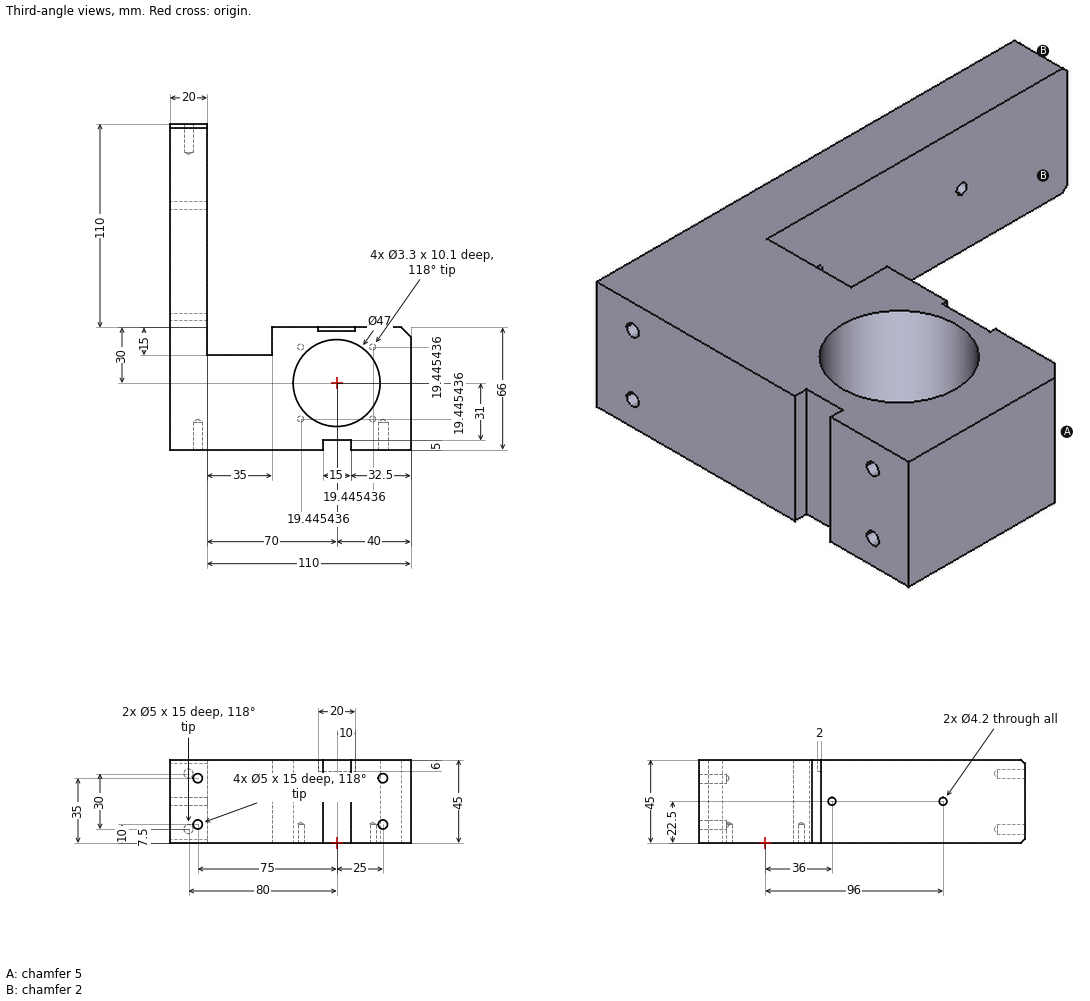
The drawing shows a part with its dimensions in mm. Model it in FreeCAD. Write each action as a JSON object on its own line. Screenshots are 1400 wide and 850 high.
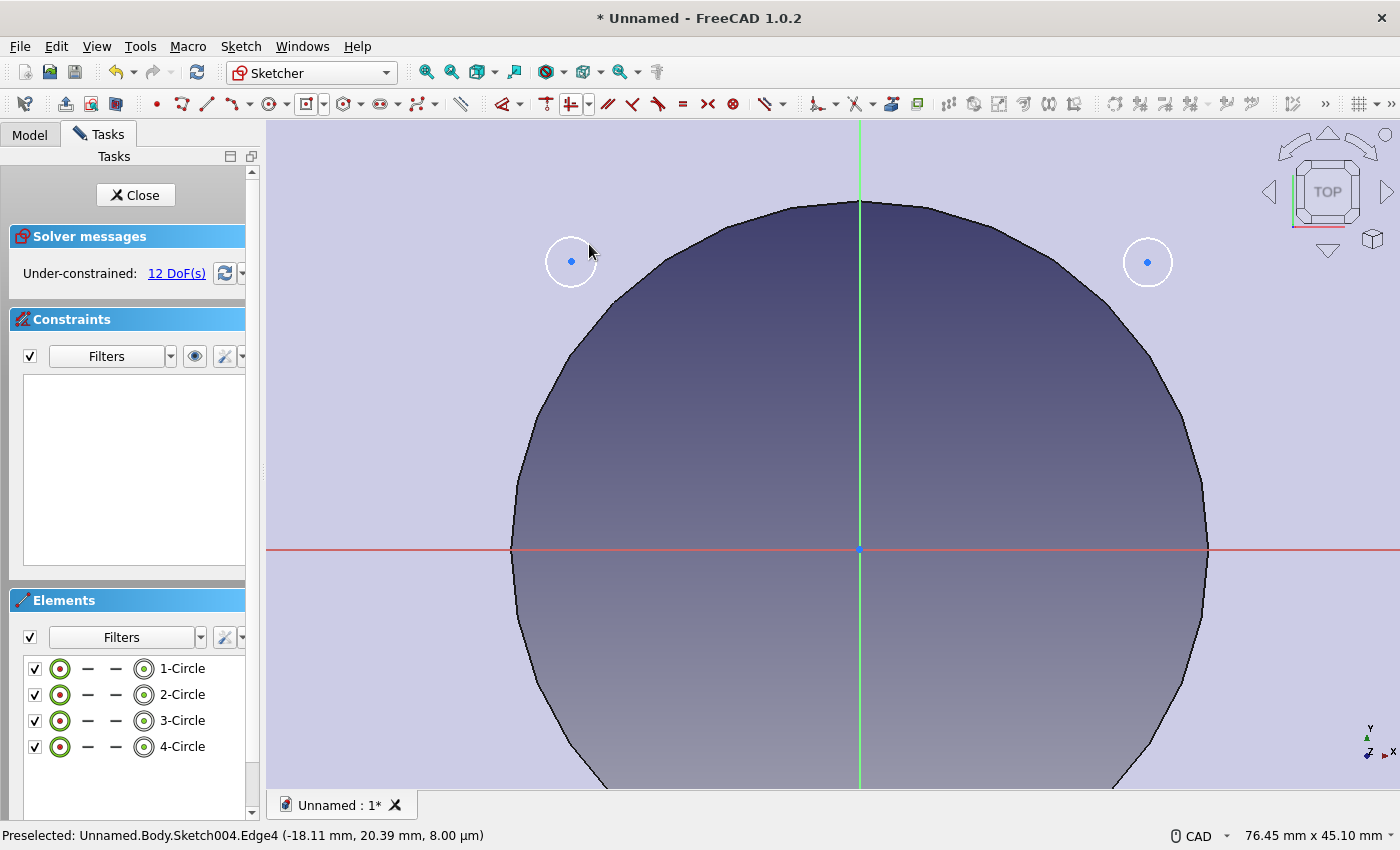
{"action": "left_click", "coordinate": [1165, 245]}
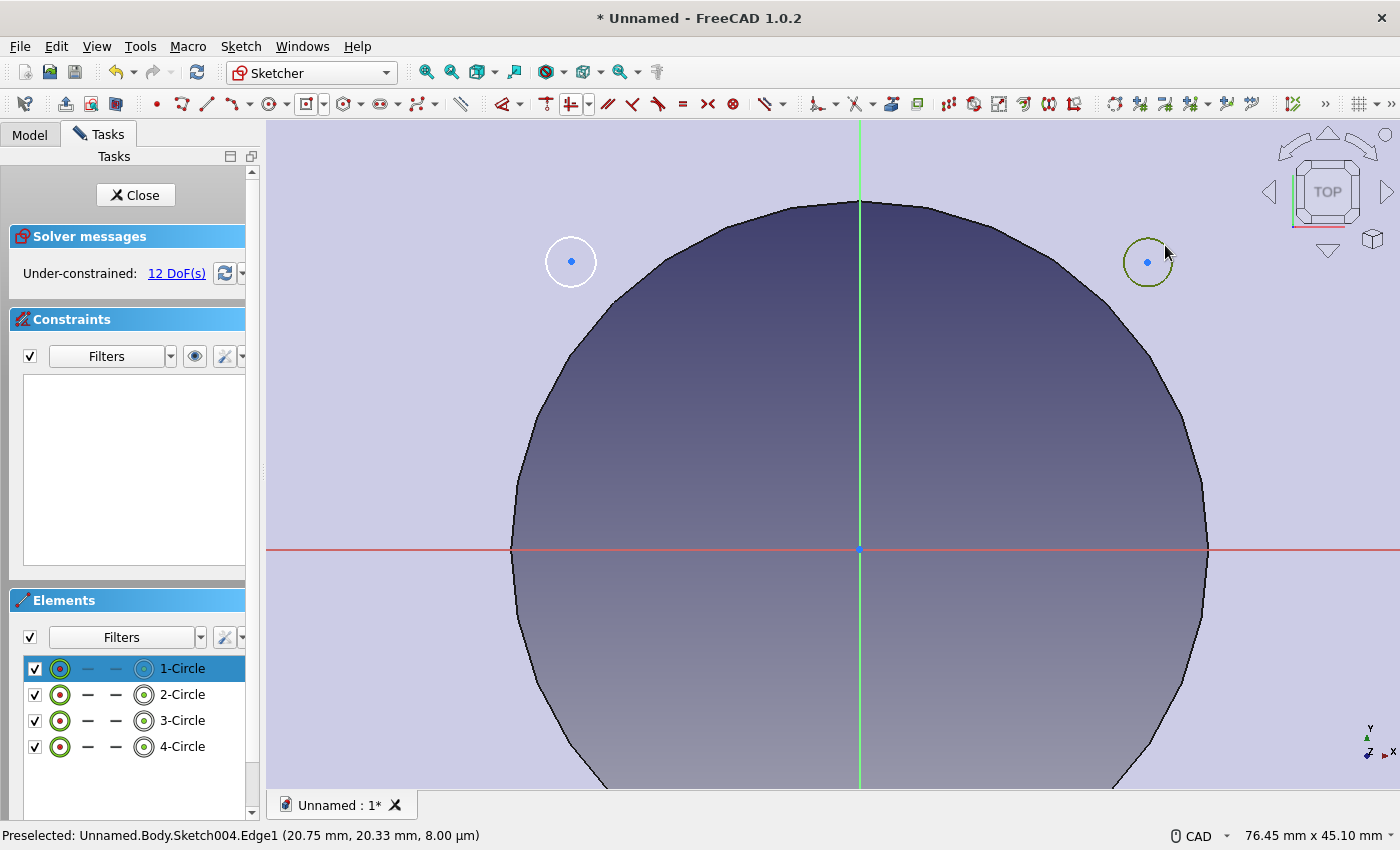
{"action": "scroll", "coordinate": [571, 261], "scroll_direction": "down", "scroll_amount": 2}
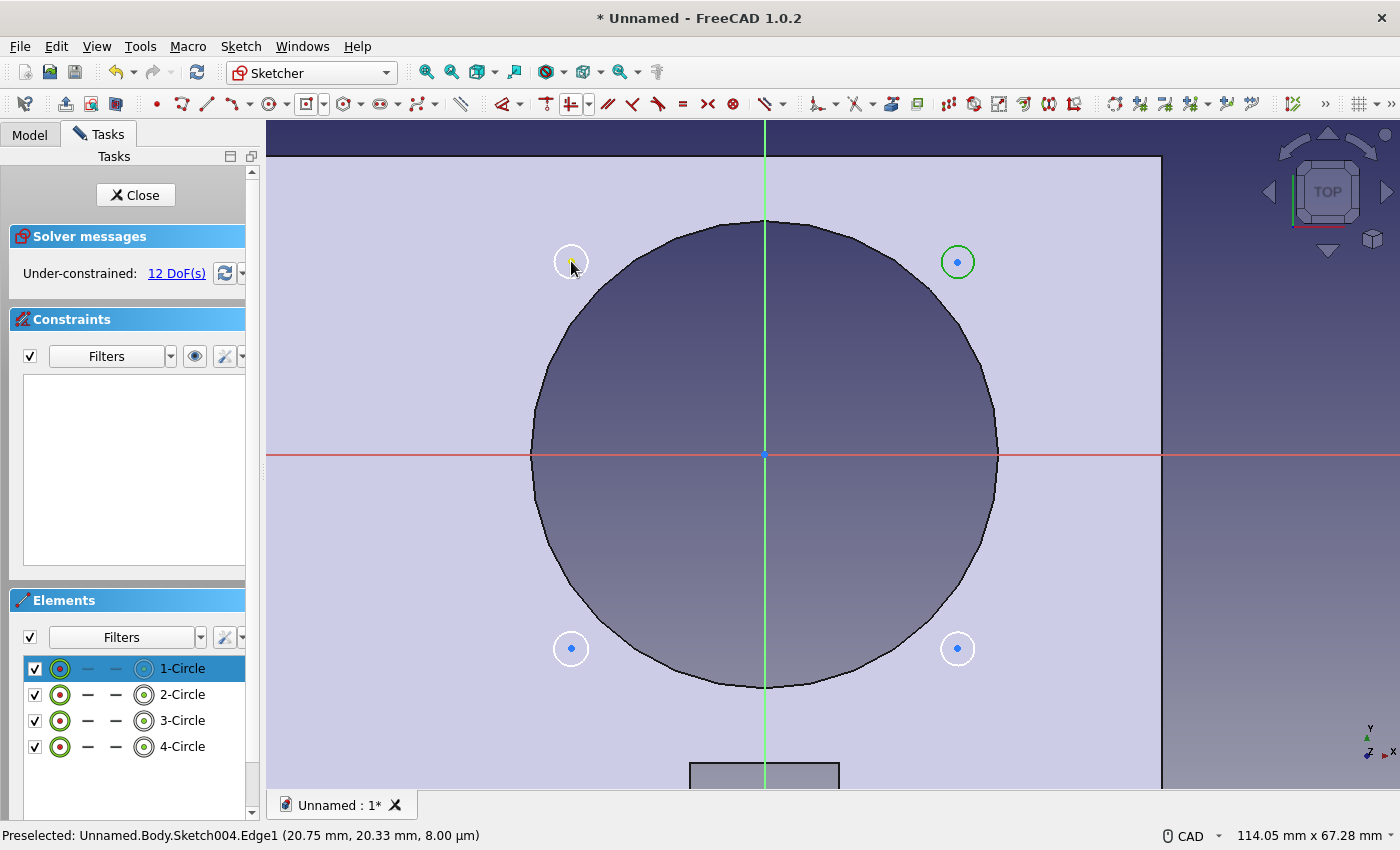
{"action": "left_click", "coordinate": [583, 637]}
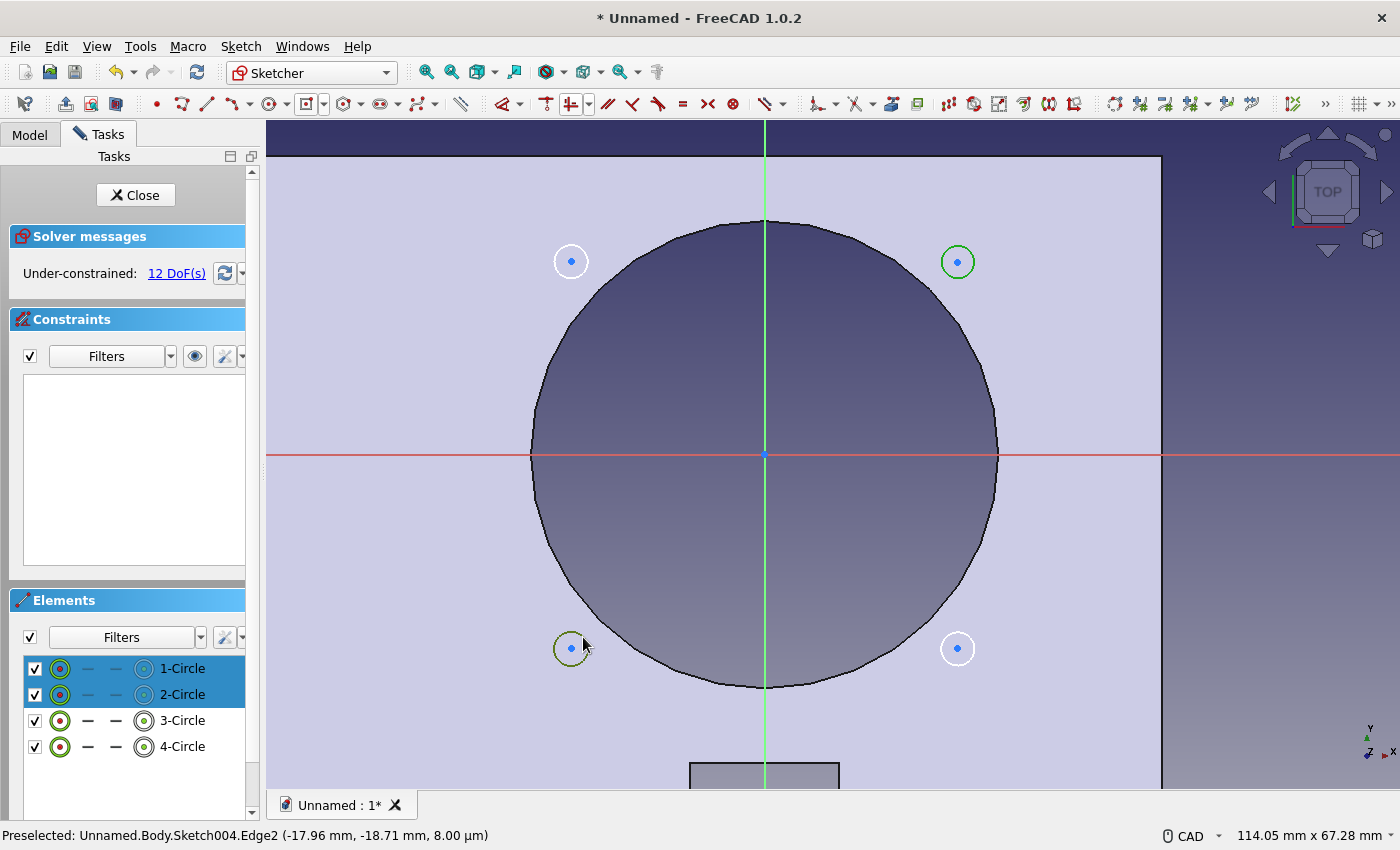
{"action": "left_click", "coordinate": [970, 637]}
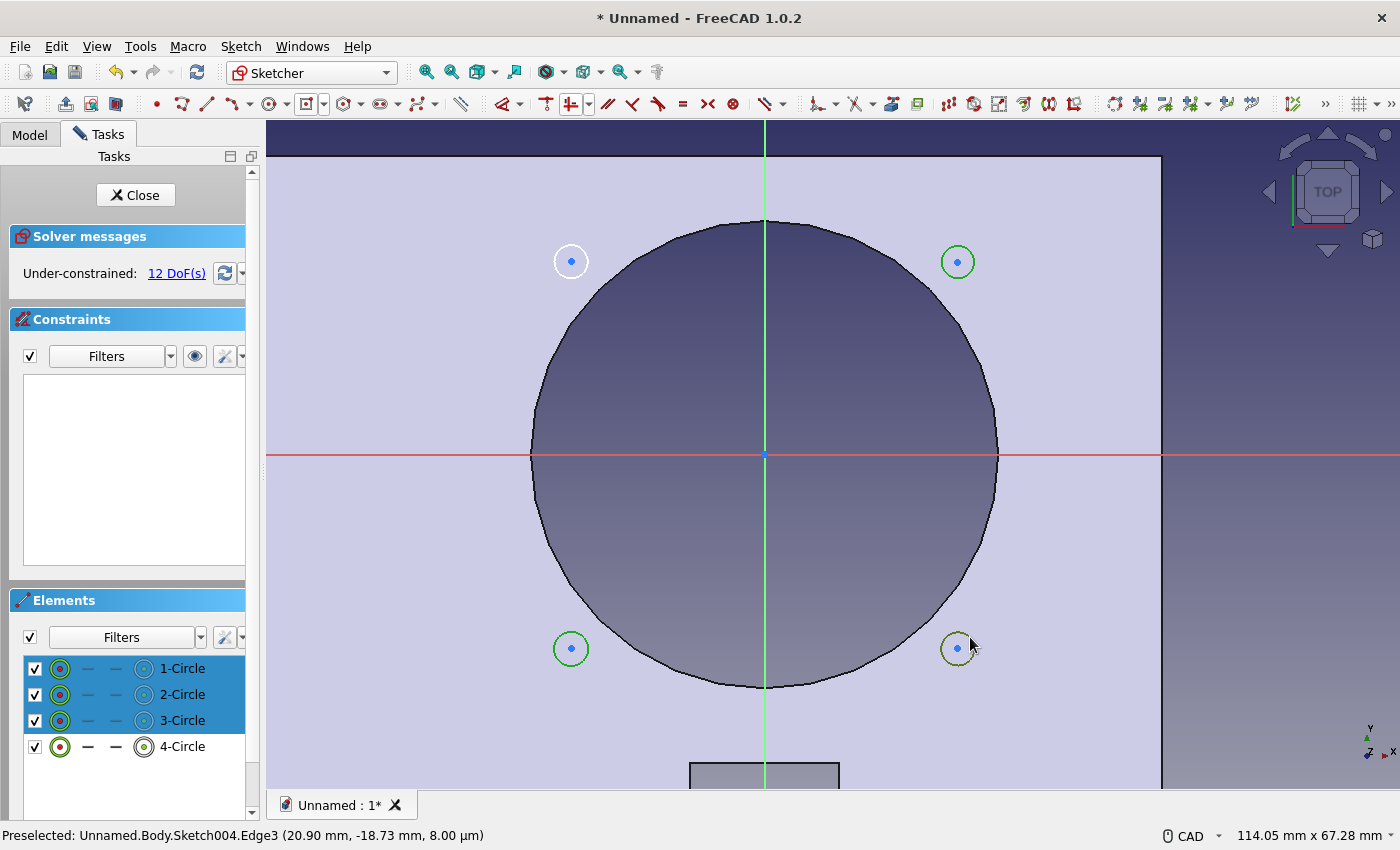
{"action": "left_click", "coordinate": [583, 250]}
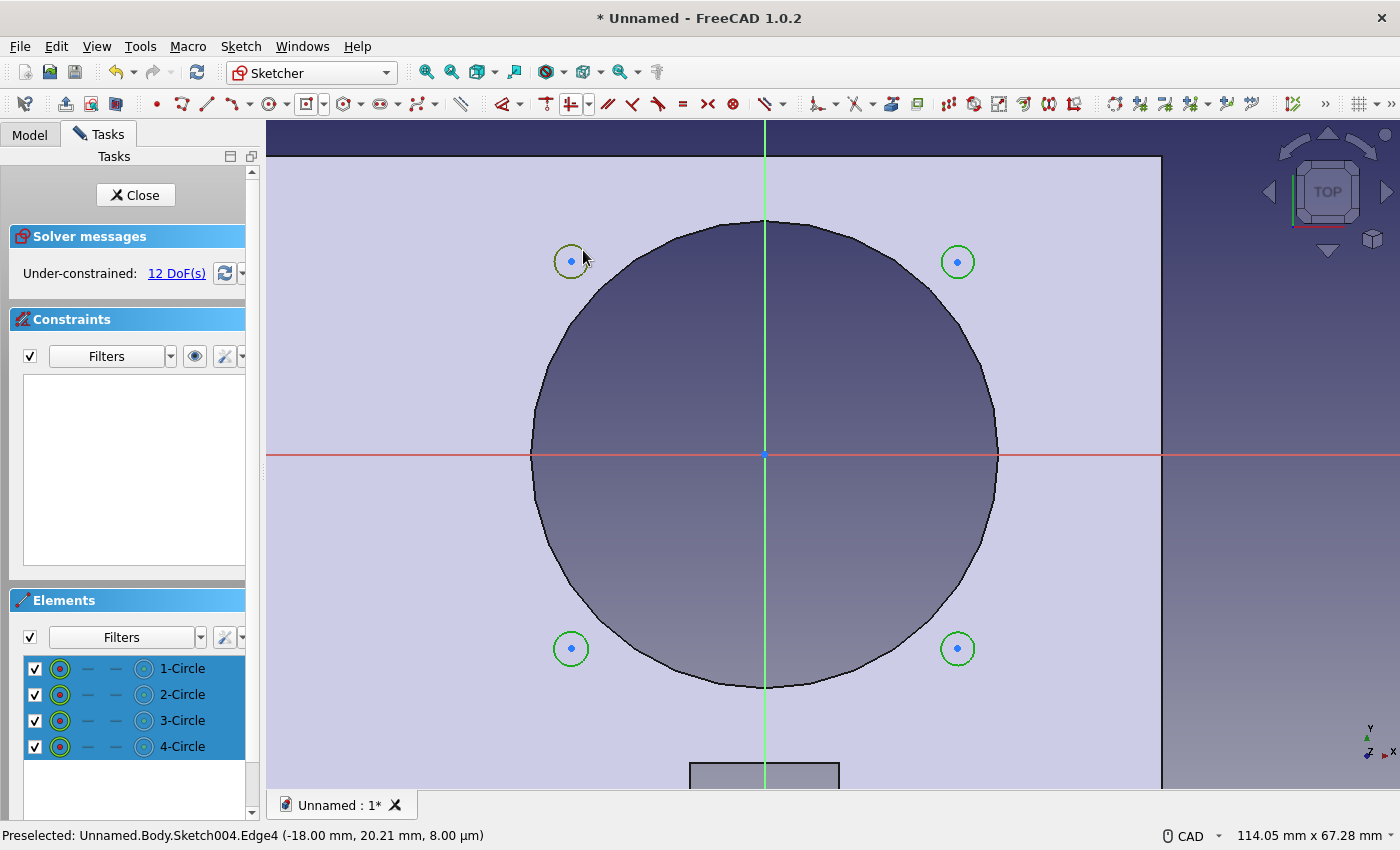
{"action": "left_click", "coordinate": [683, 104]}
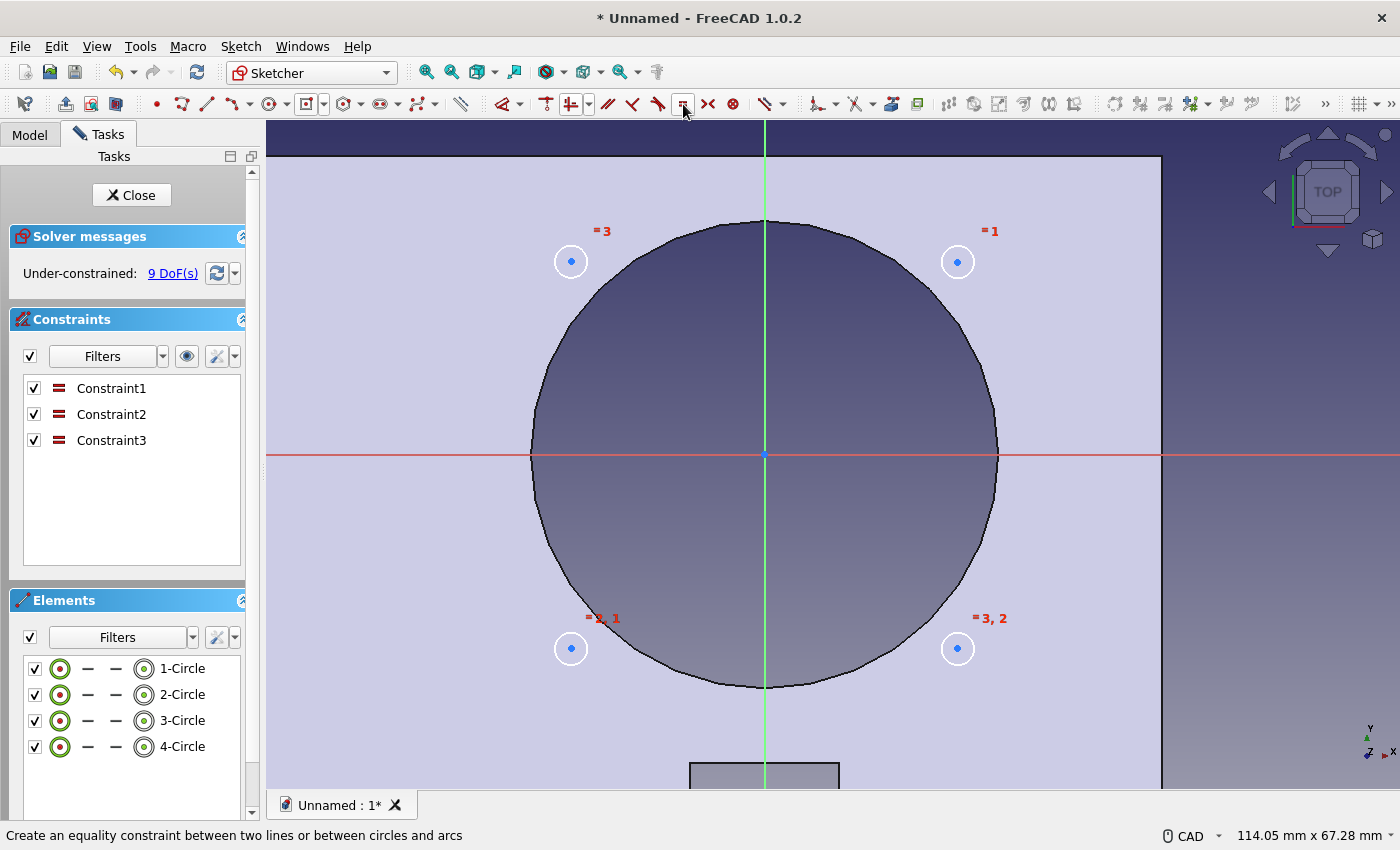
{"action": "left_click", "coordinate": [958, 262]}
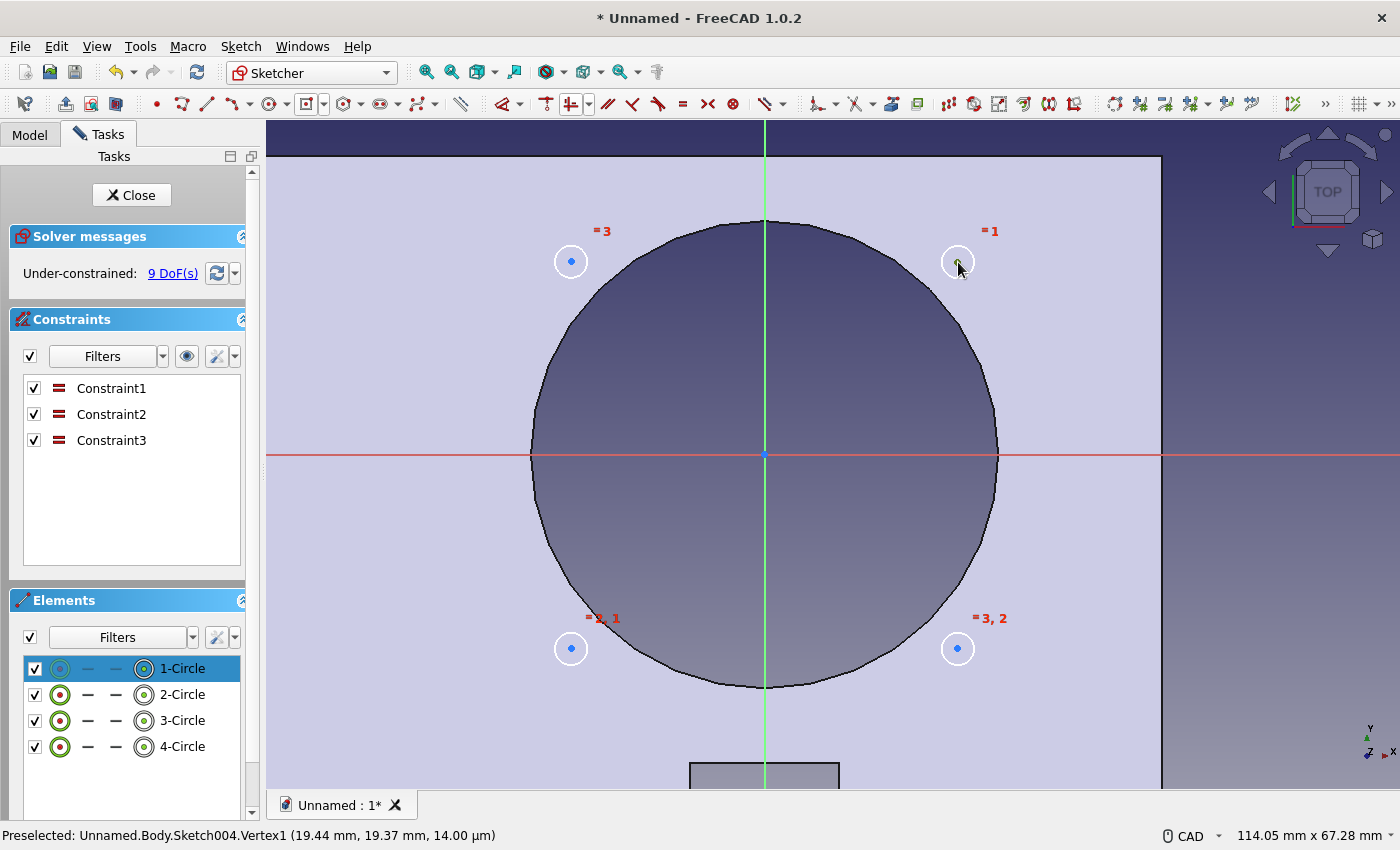
{"action": "left_click", "coordinate": [958, 649]}